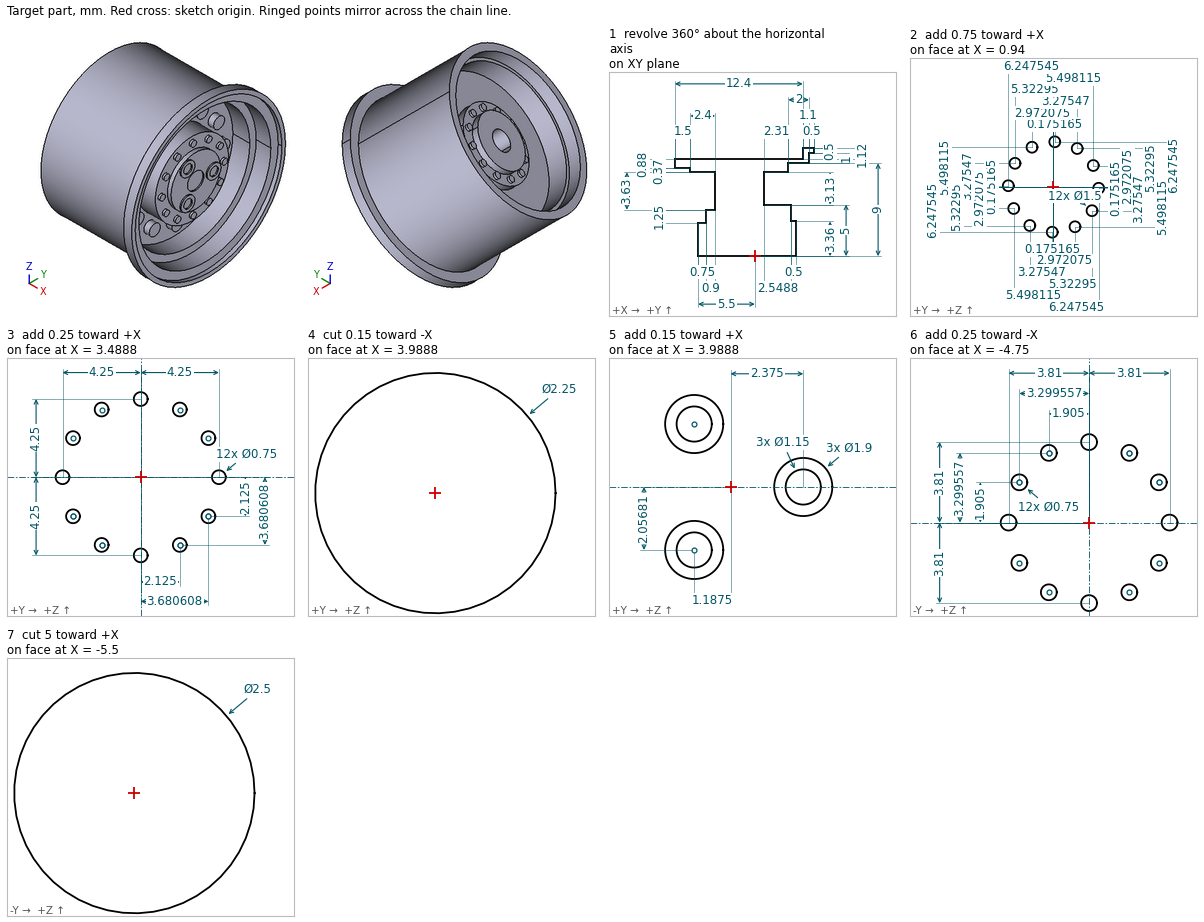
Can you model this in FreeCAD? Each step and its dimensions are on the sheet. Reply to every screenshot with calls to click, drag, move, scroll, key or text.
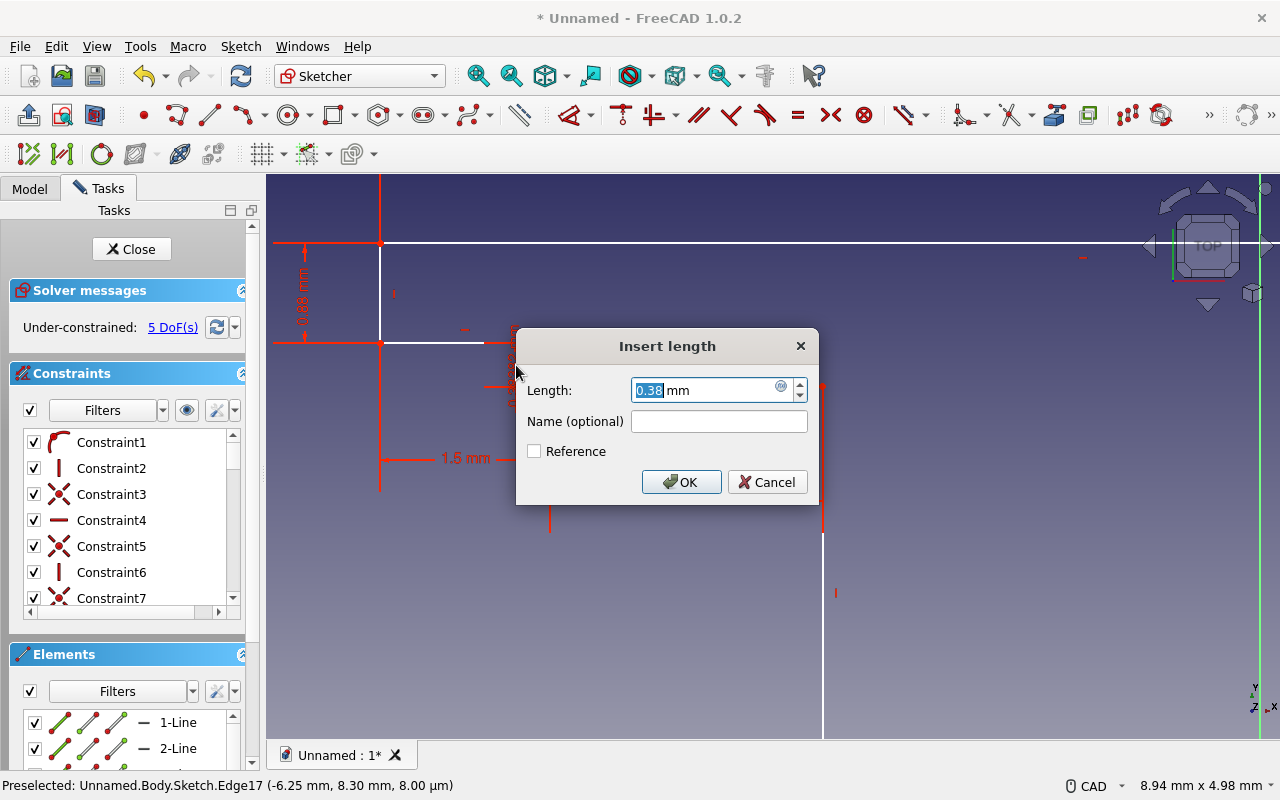
text(0.37)
key(Return)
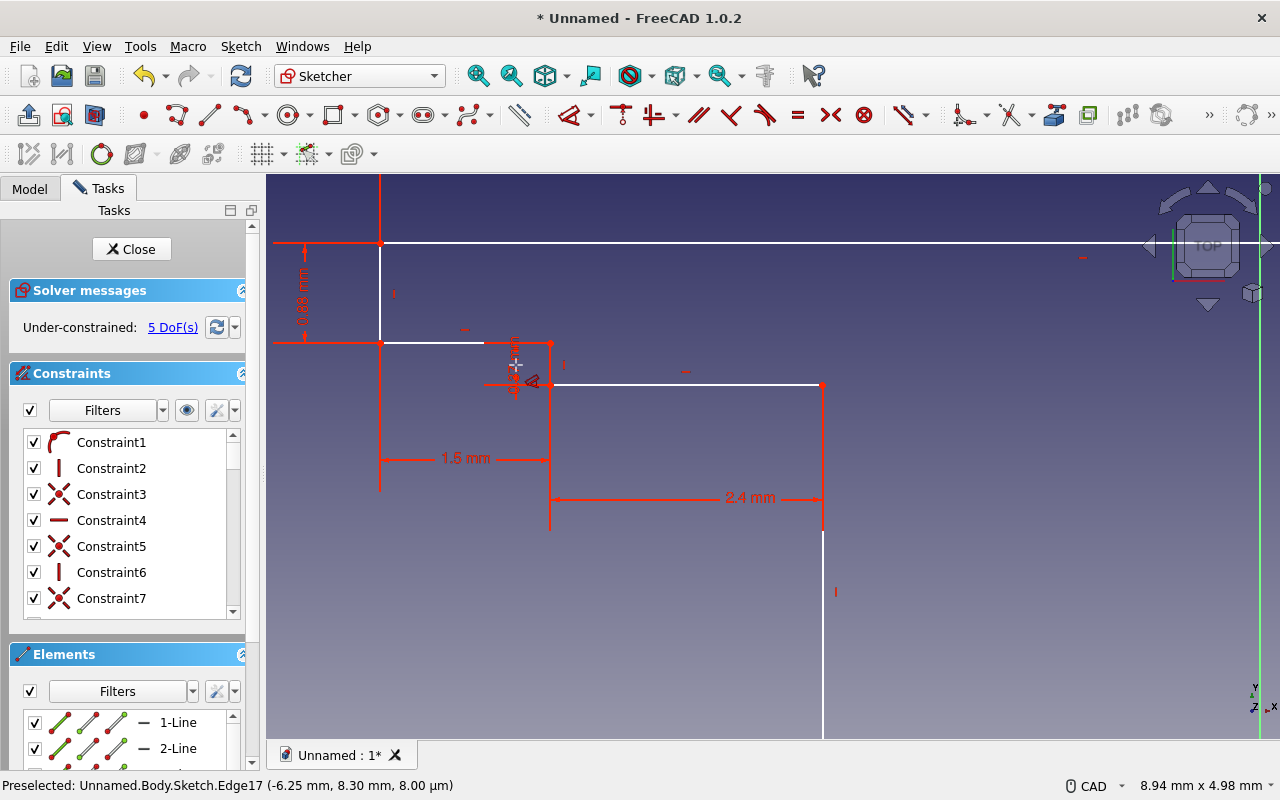
click(823, 509)
click(789, 548)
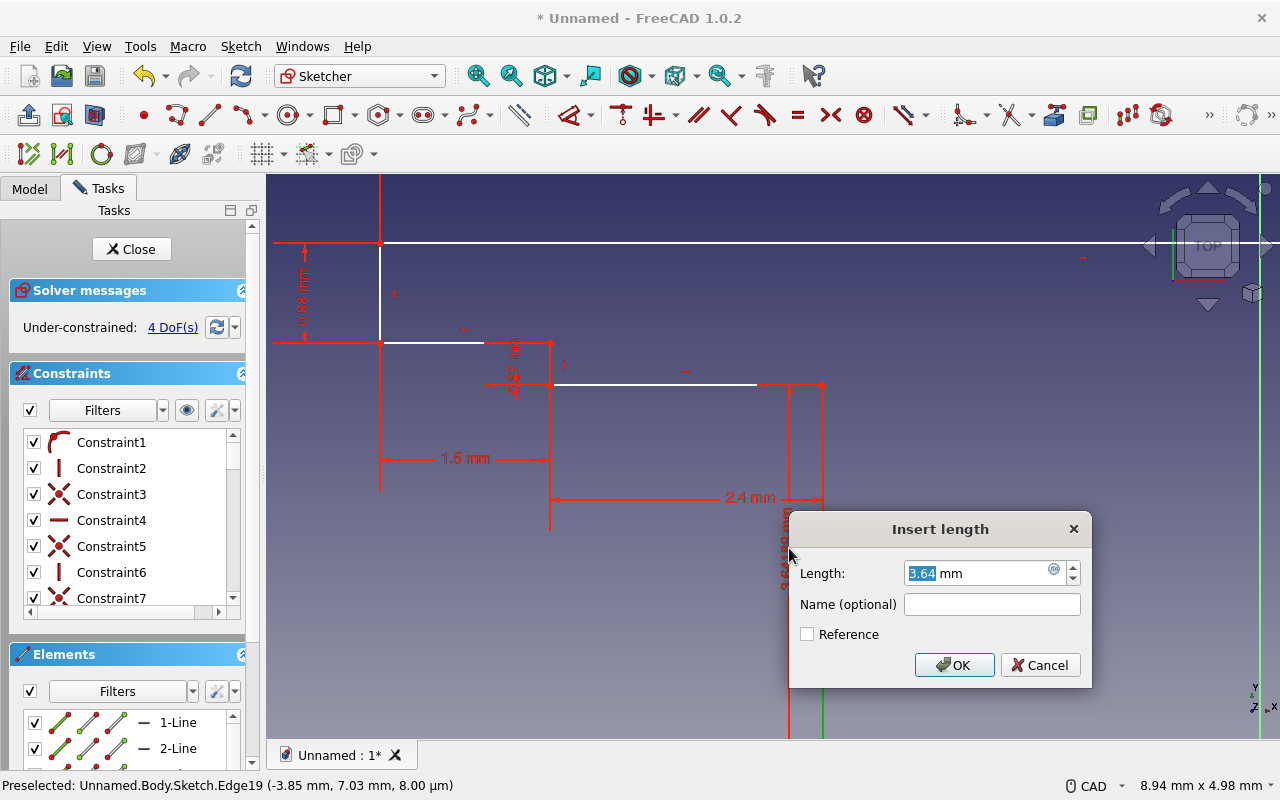
text(3.63)
key(Return)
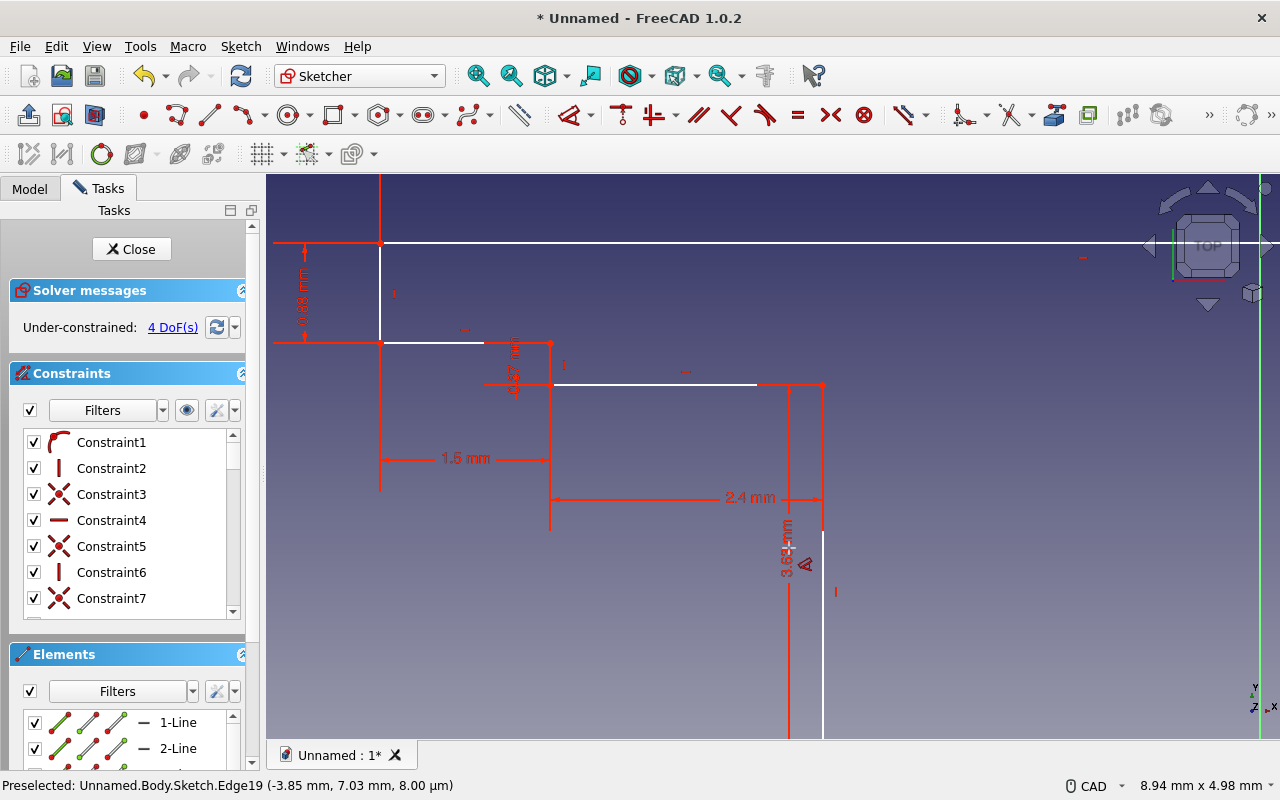
scroll(514, 346, down, 6)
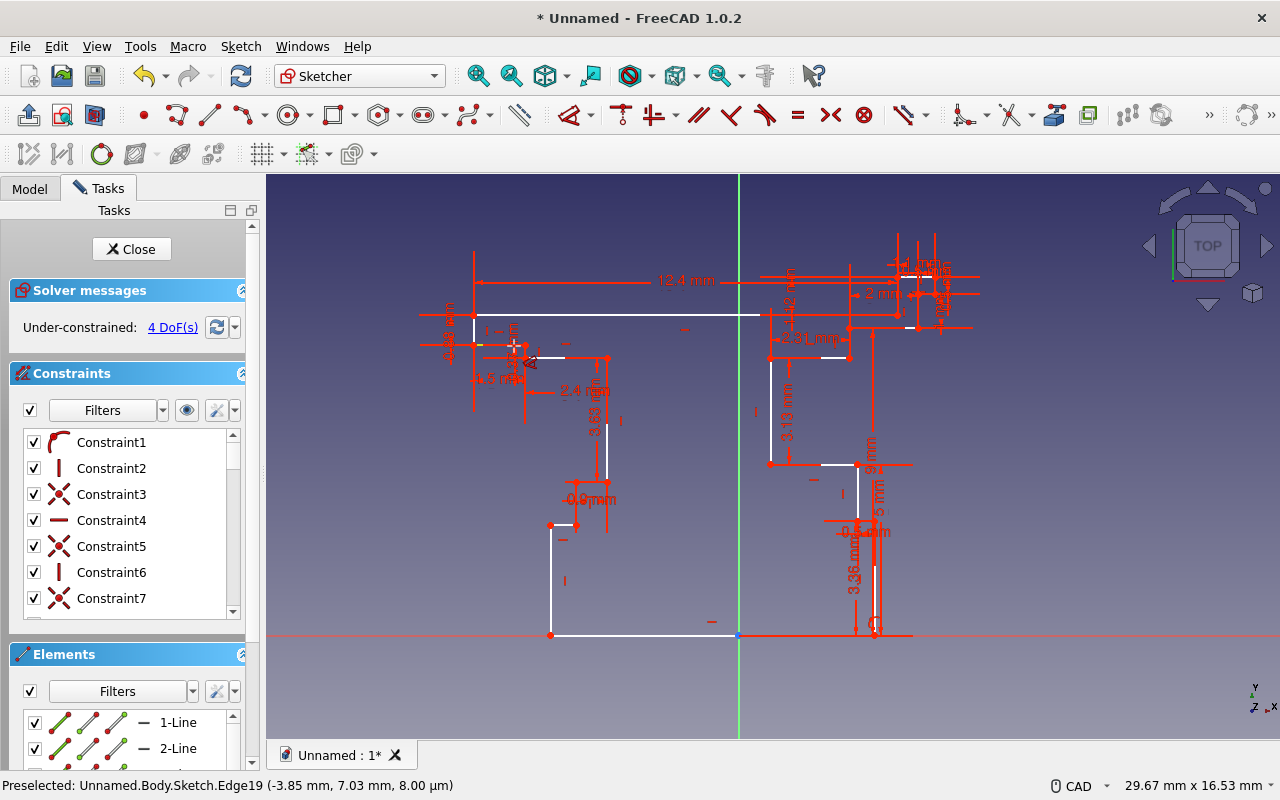
click(576, 495)
click(518, 504)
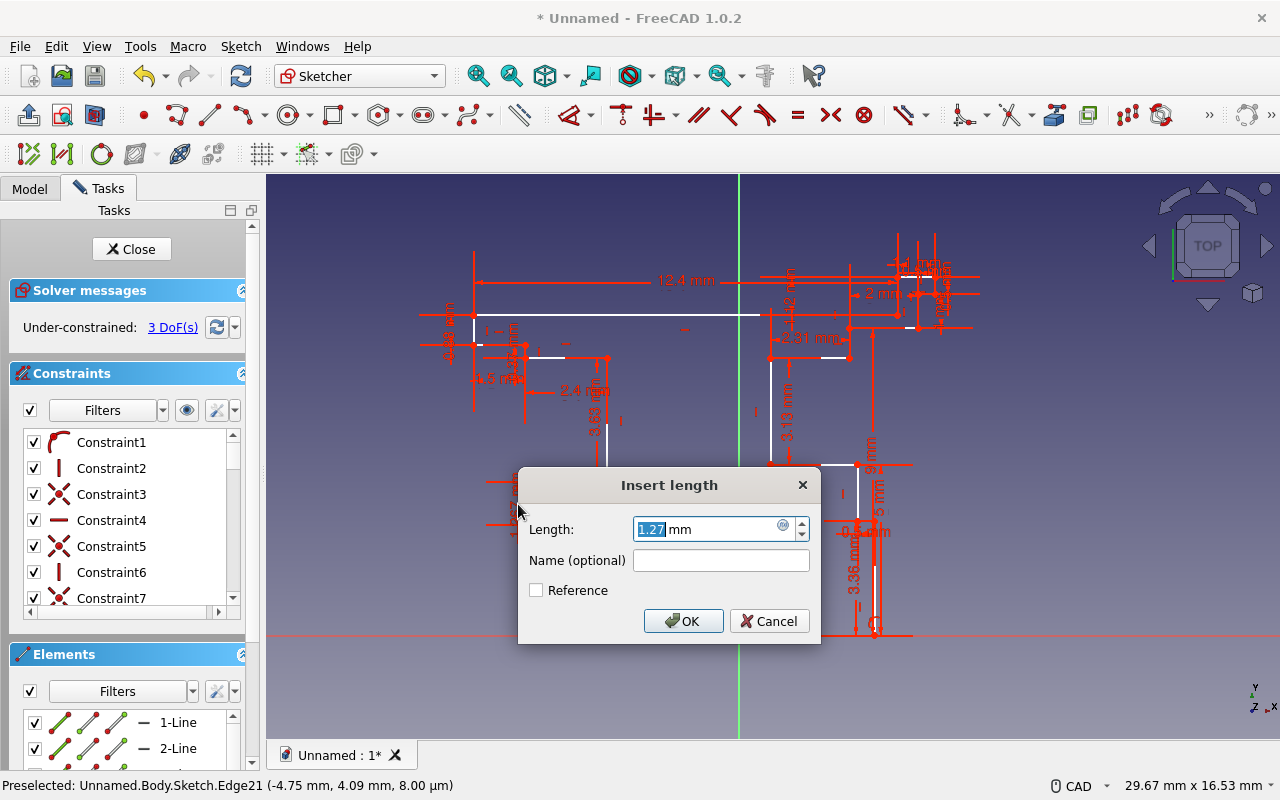
text(1.25)
key(Return)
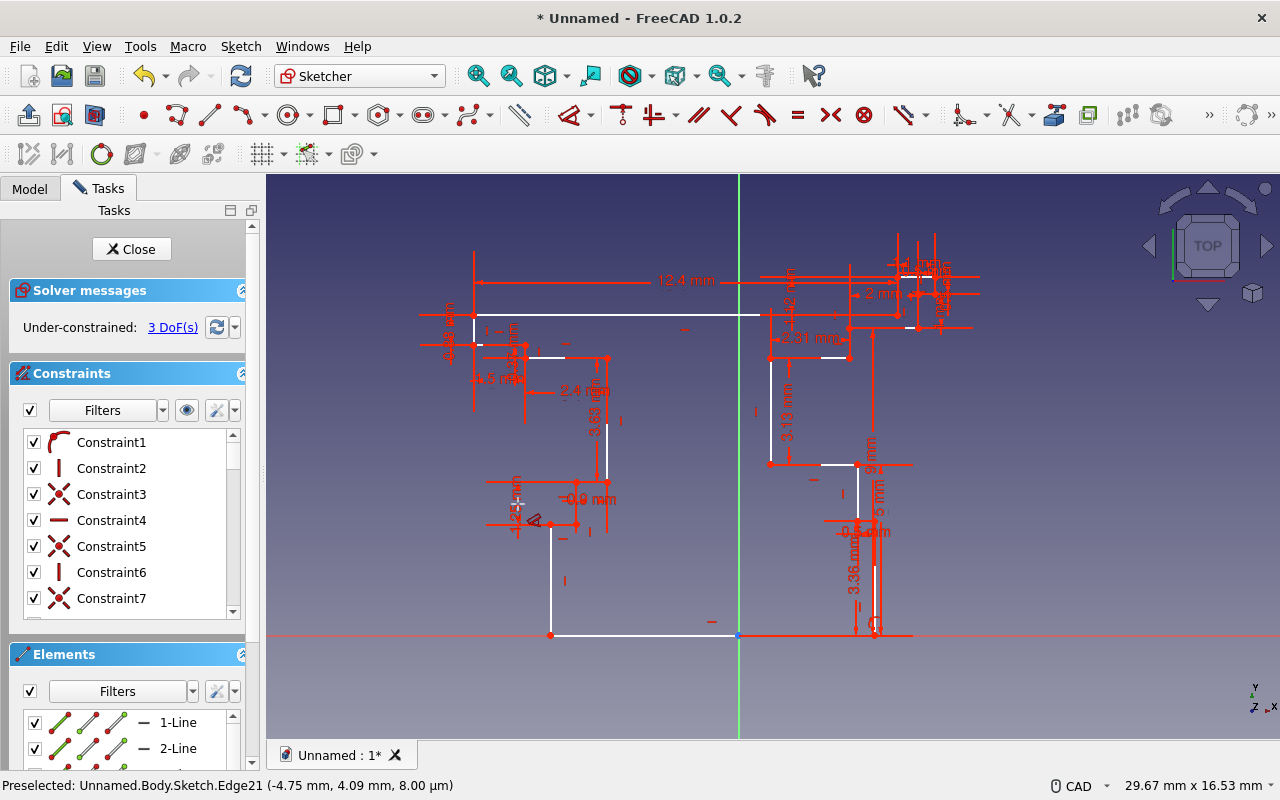
scroll(566, 525, up, 3)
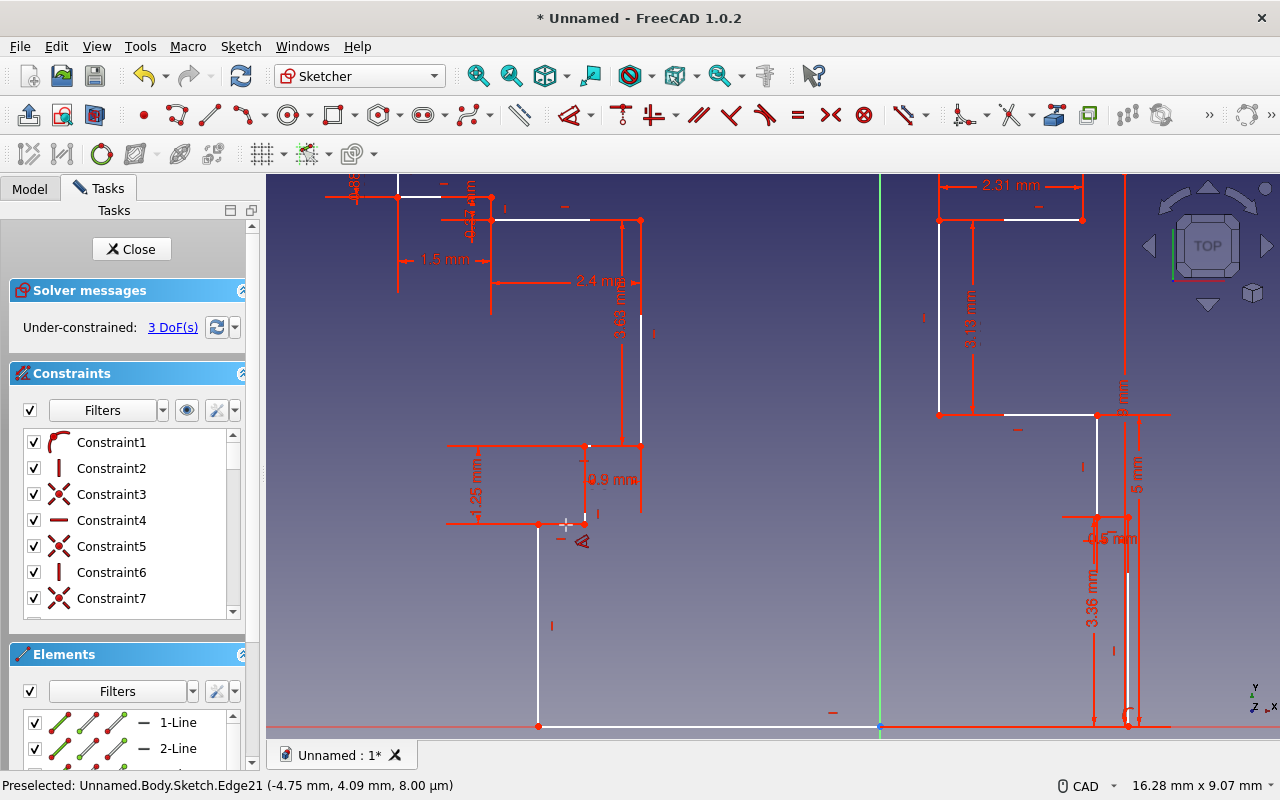
click(566, 524)
click(561, 558)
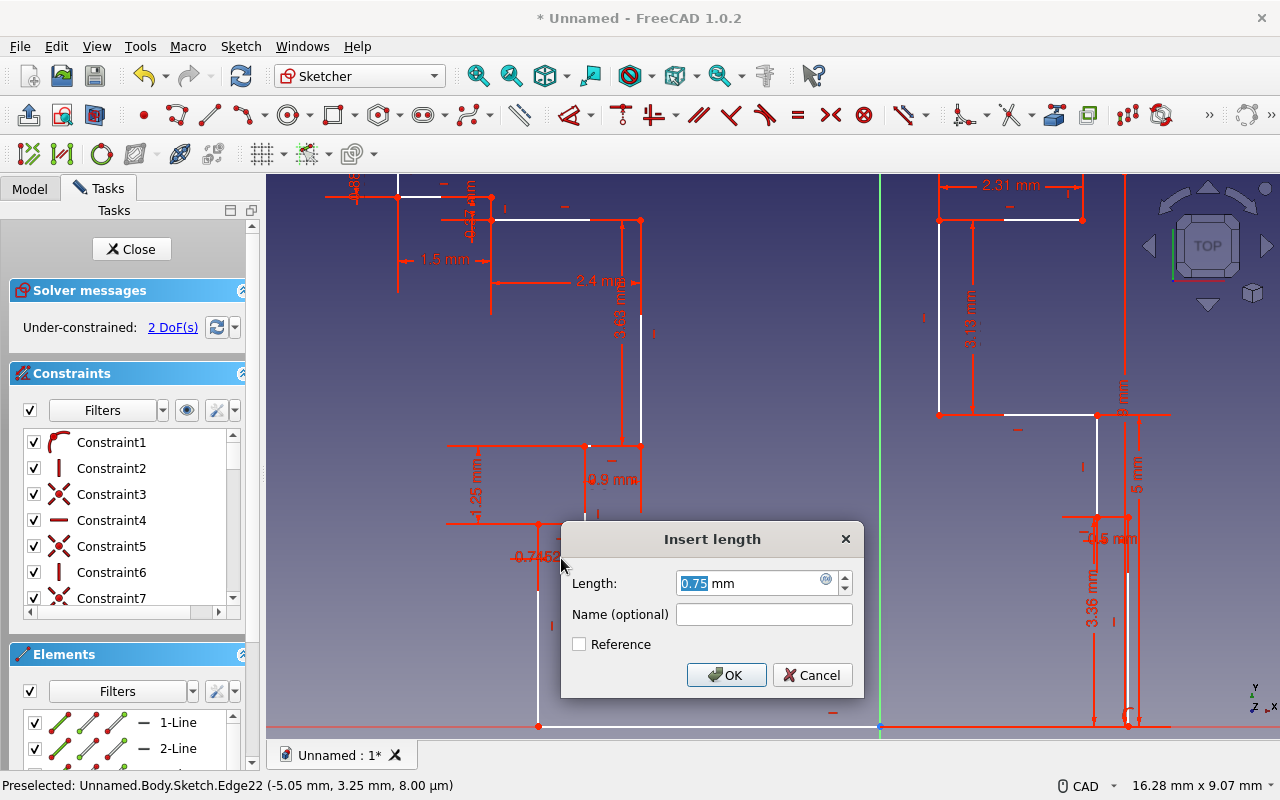
text(0.75)
key(Return)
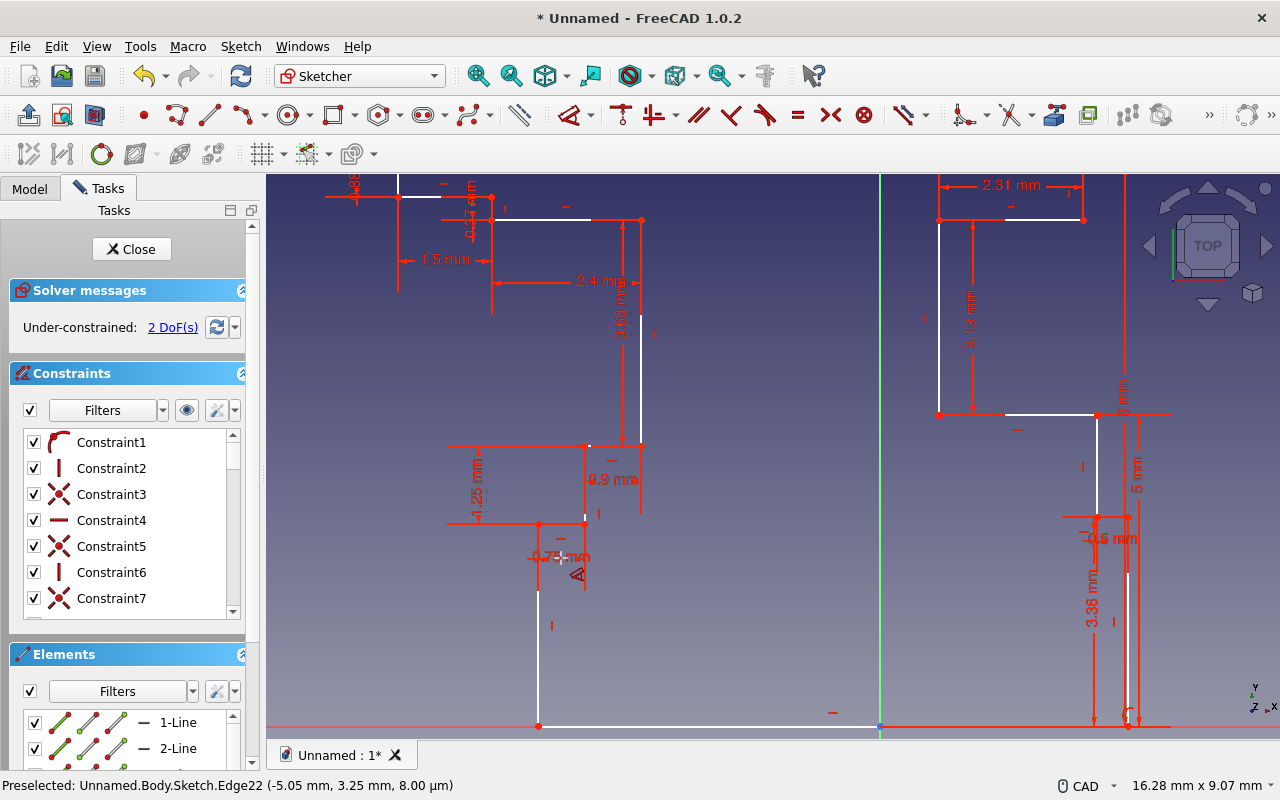
click(538, 524)
click(709, 490)